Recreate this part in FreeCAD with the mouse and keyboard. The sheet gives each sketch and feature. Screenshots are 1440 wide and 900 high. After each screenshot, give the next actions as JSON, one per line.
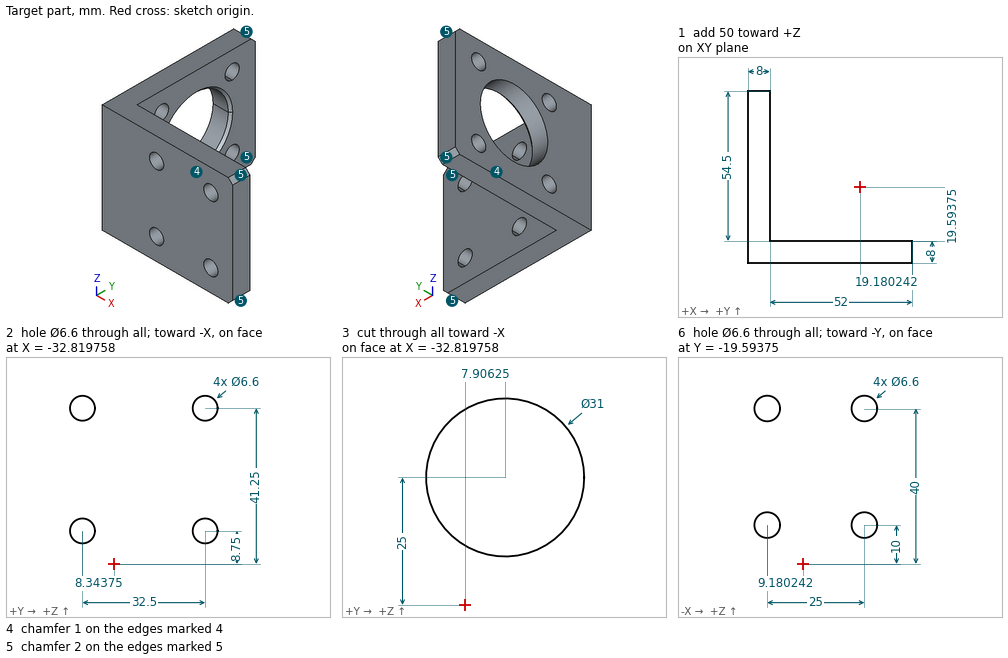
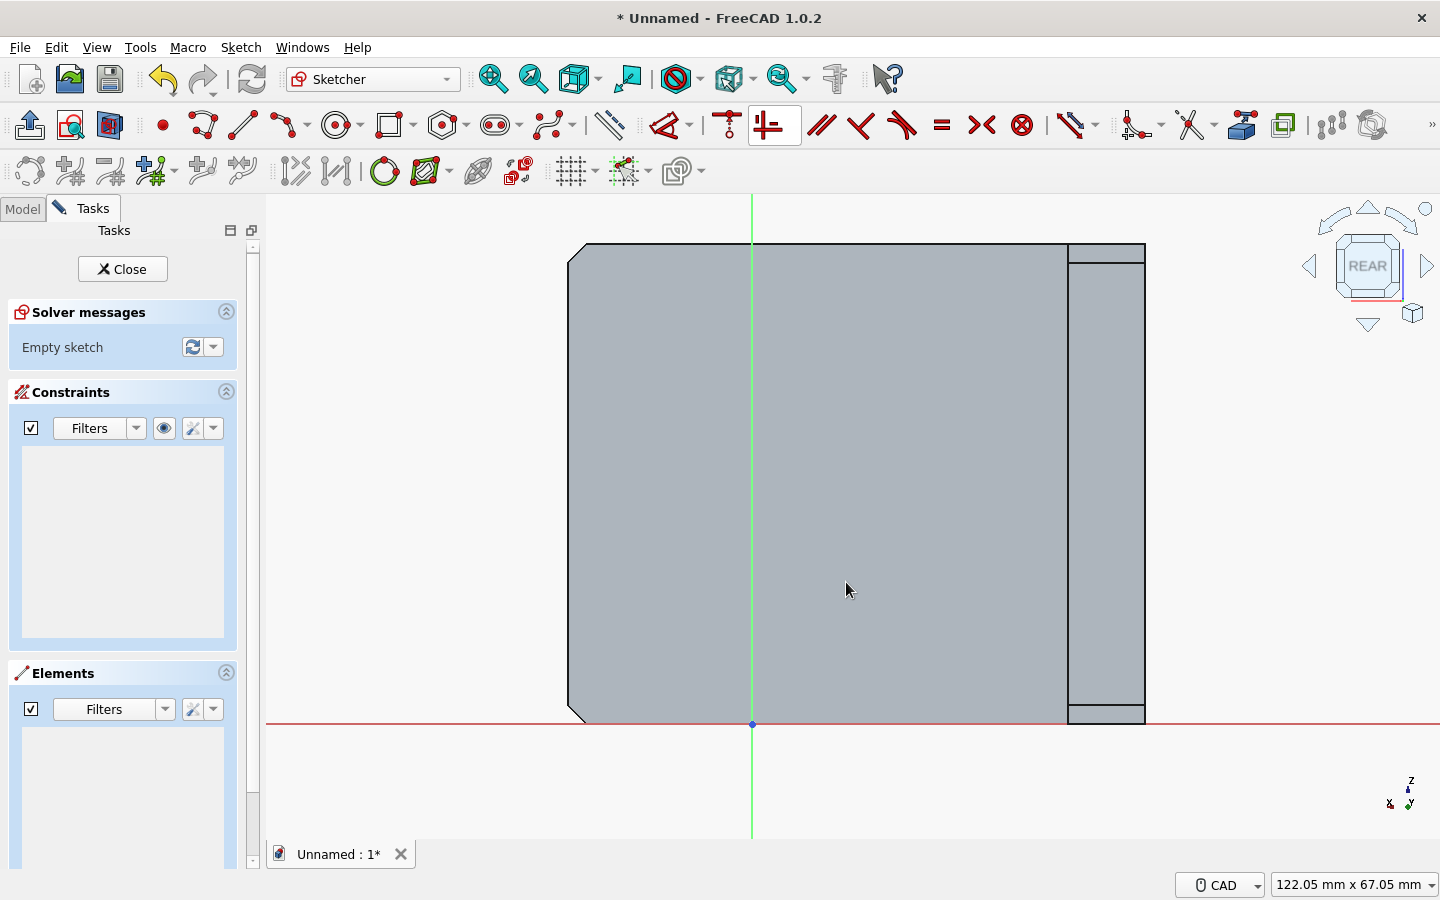
{"action": "left_click", "coordinate": [336, 126]}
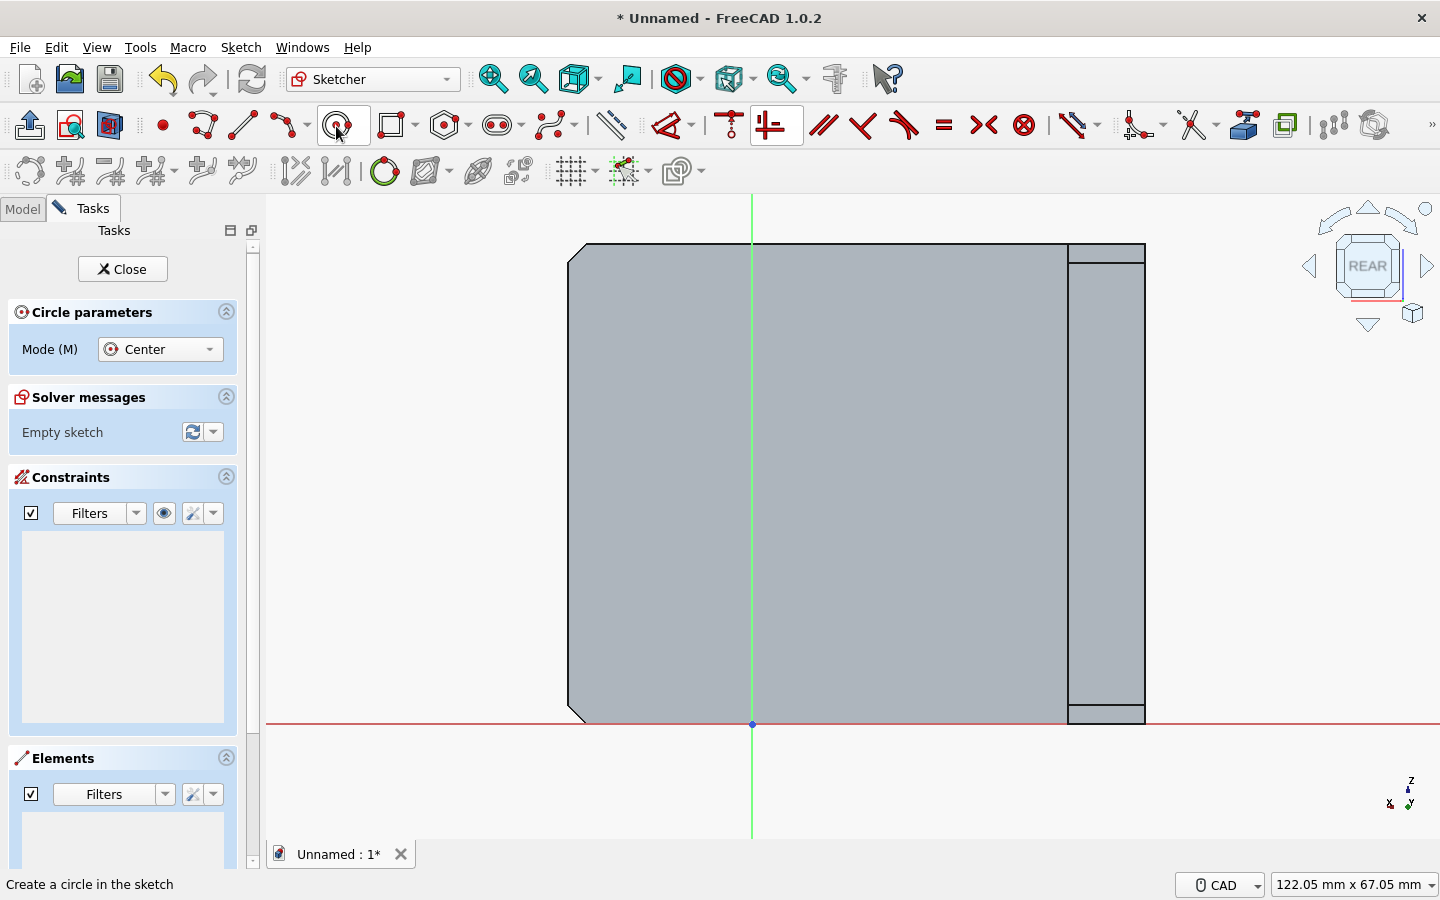
{"action": "left_click", "coordinate": [904, 340]}
{"action": "mouse_move", "coordinate": [927, 317]}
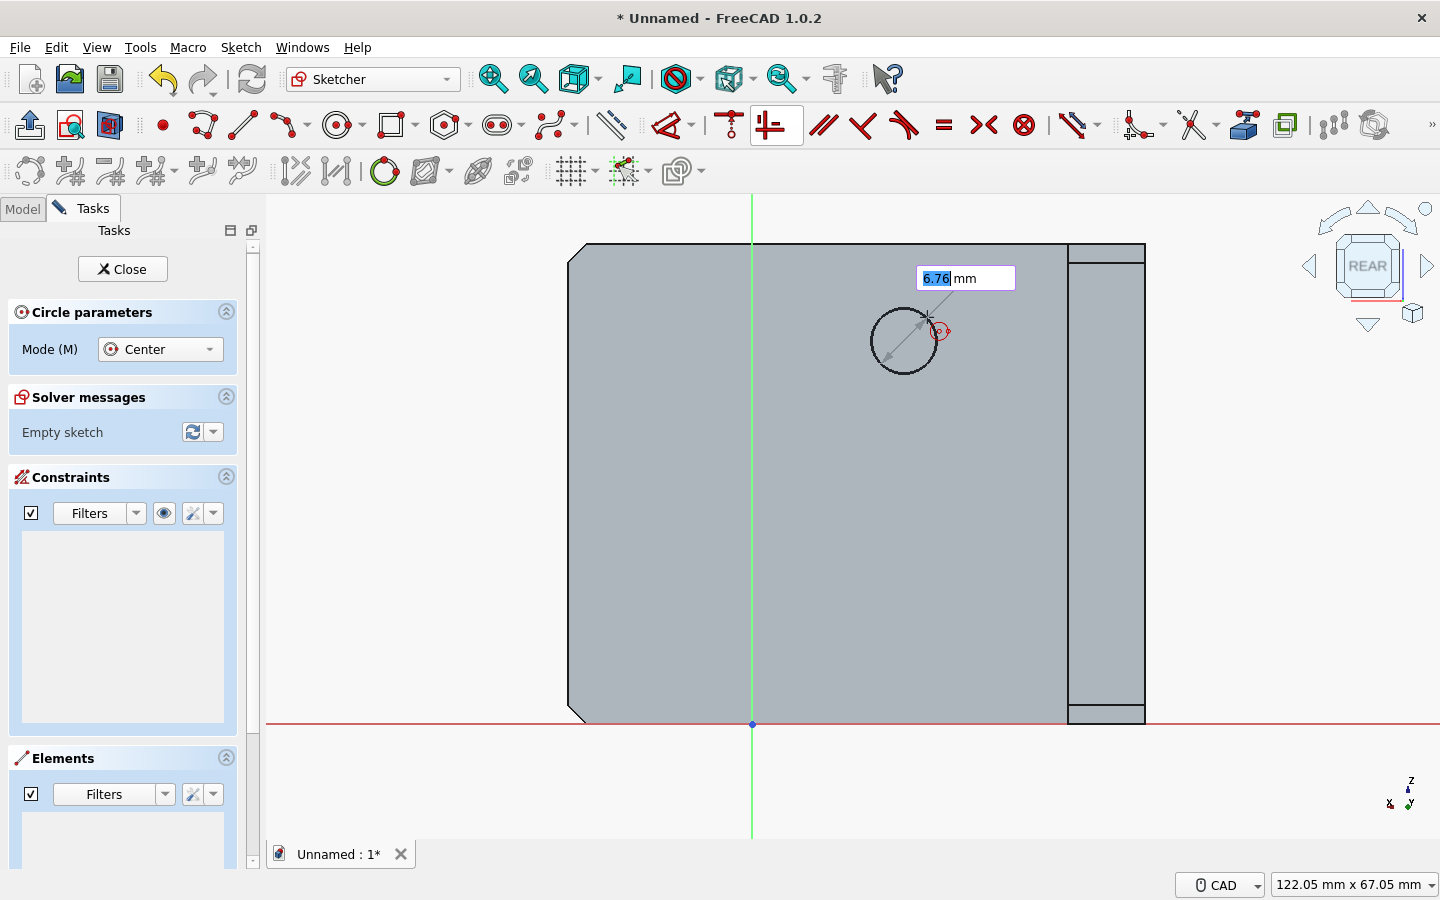
{"action": "type", "text": "6.6"}
{"action": "key", "text": "Return"}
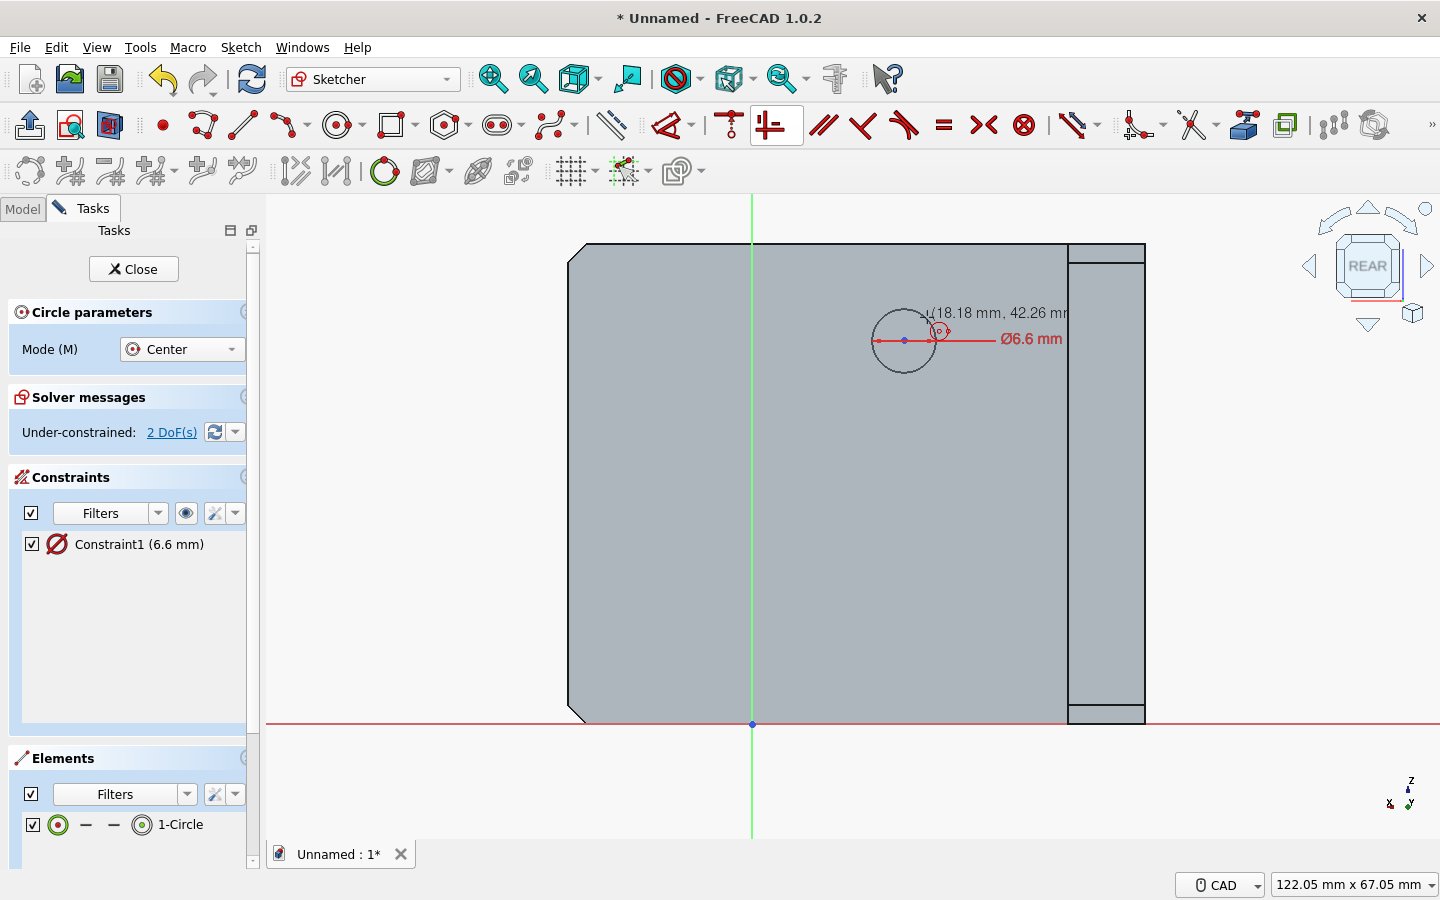
{"action": "left_click", "coordinate": [904, 628]}
{"action": "mouse_move", "coordinate": [927, 606]}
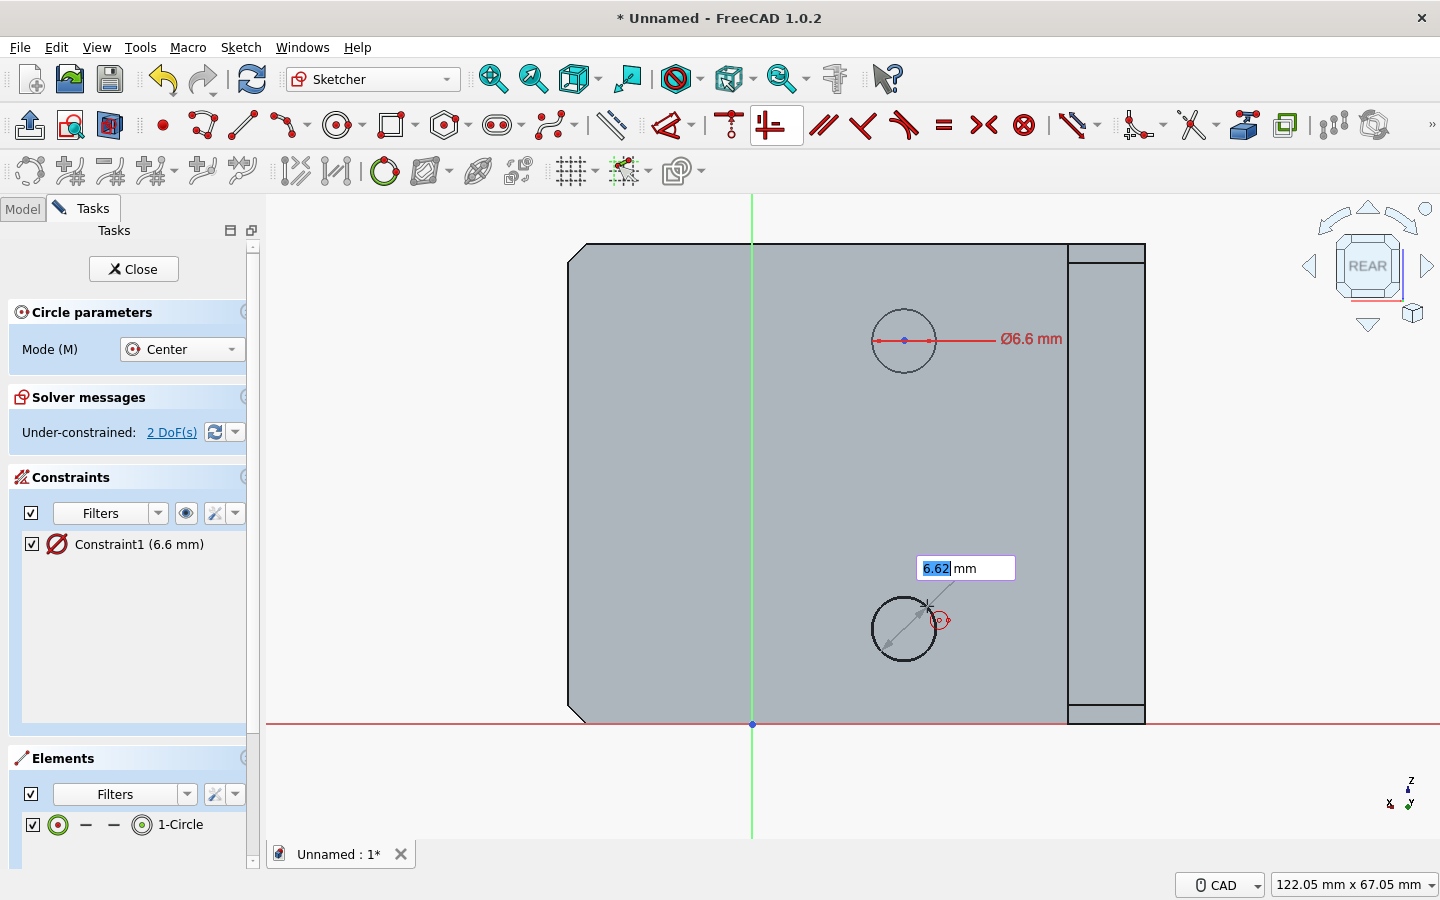
{"action": "type", "text": "6.6"}
{"action": "key", "text": "Return"}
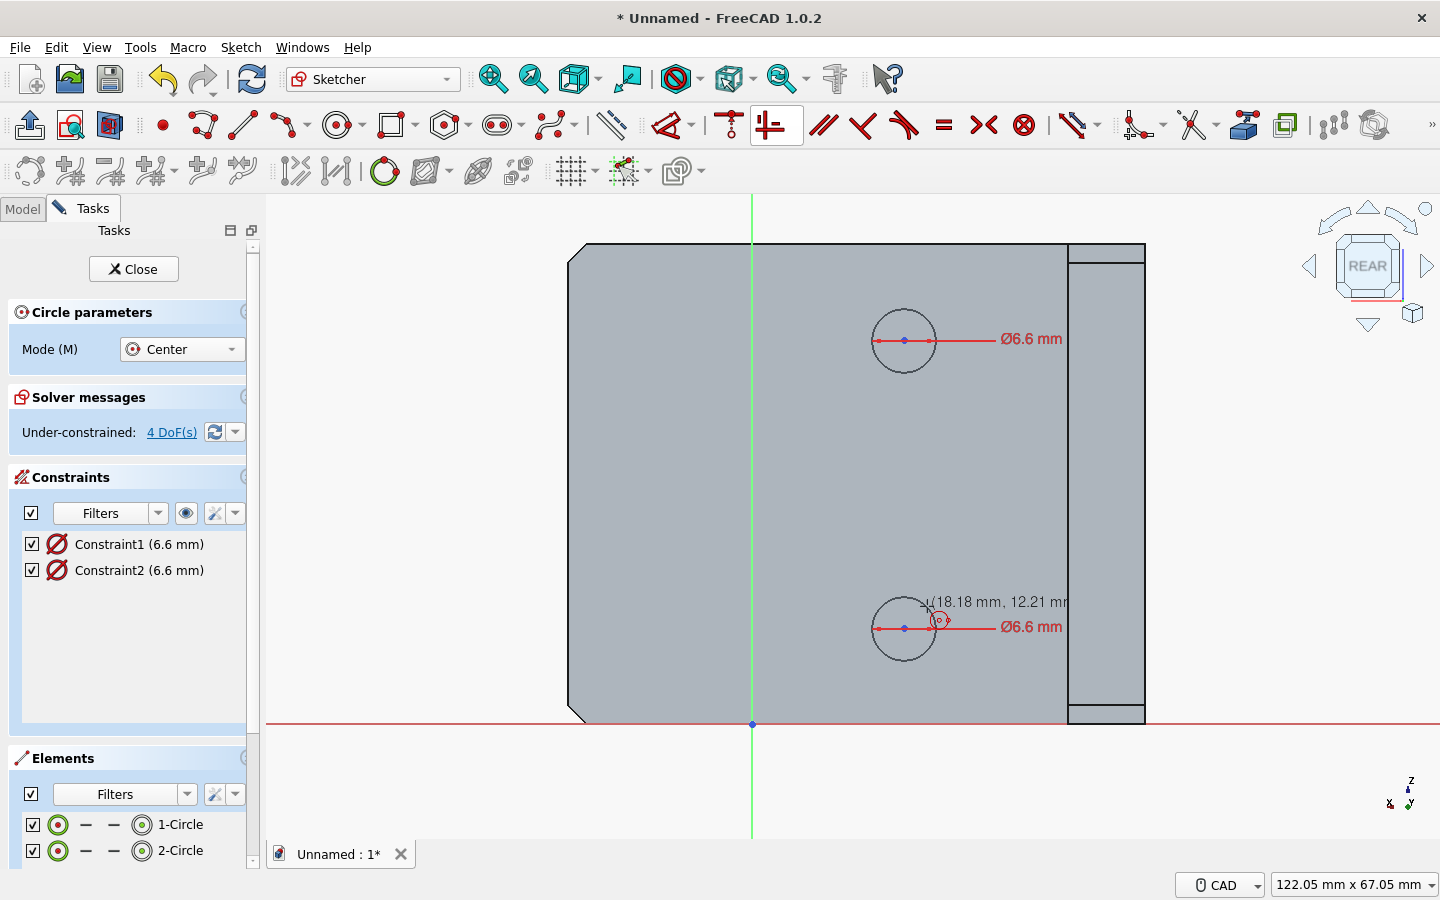
{"action": "left_click", "coordinate": [664, 628]}
{"action": "mouse_move", "coordinate": [686, 606]}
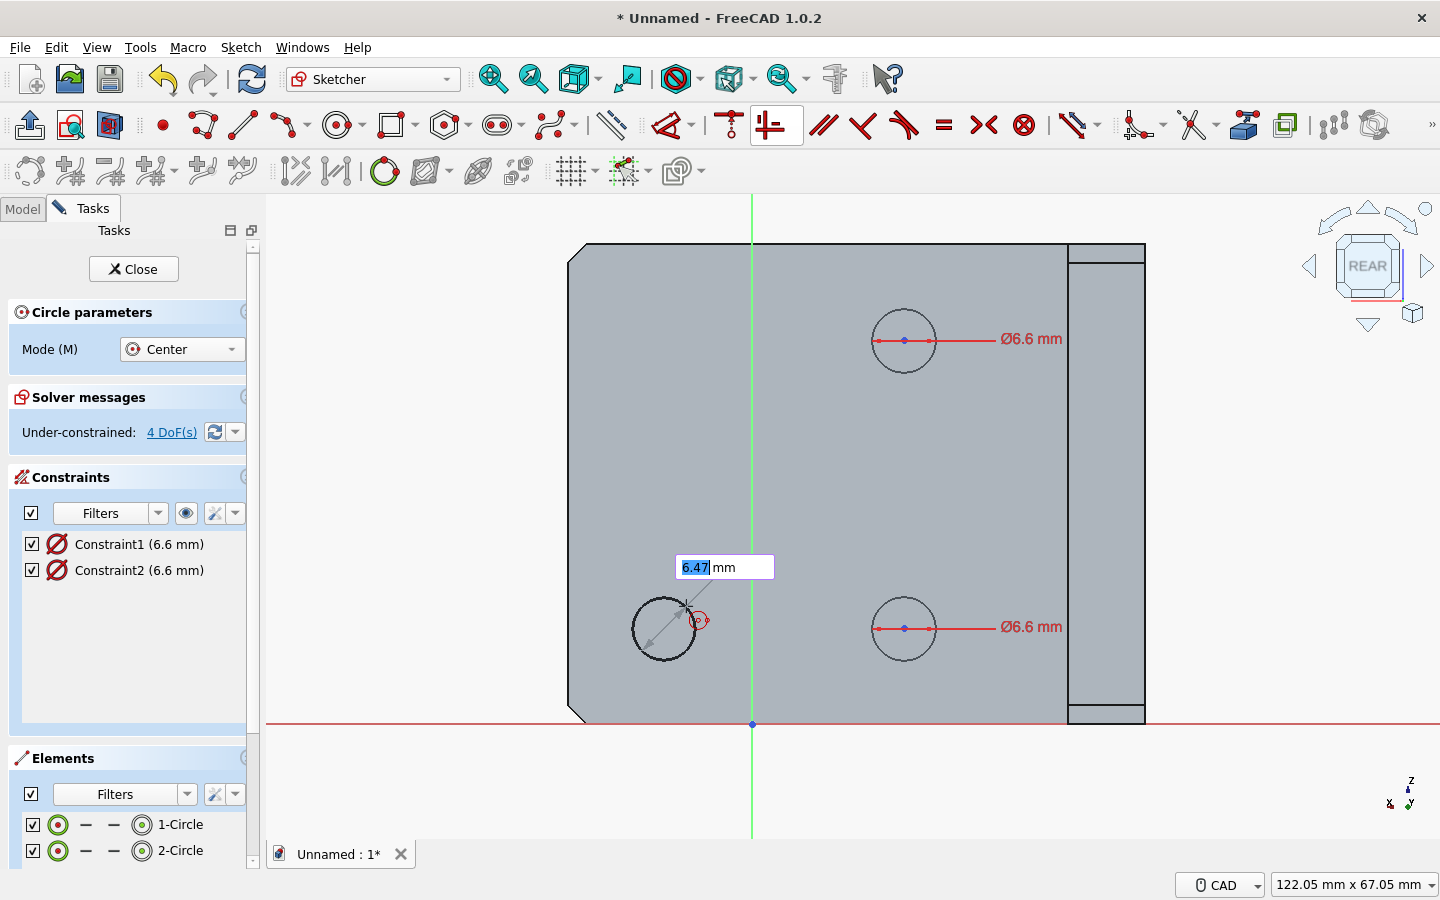
{"action": "type", "text": "6.6"}
{"action": "key", "text": "Return"}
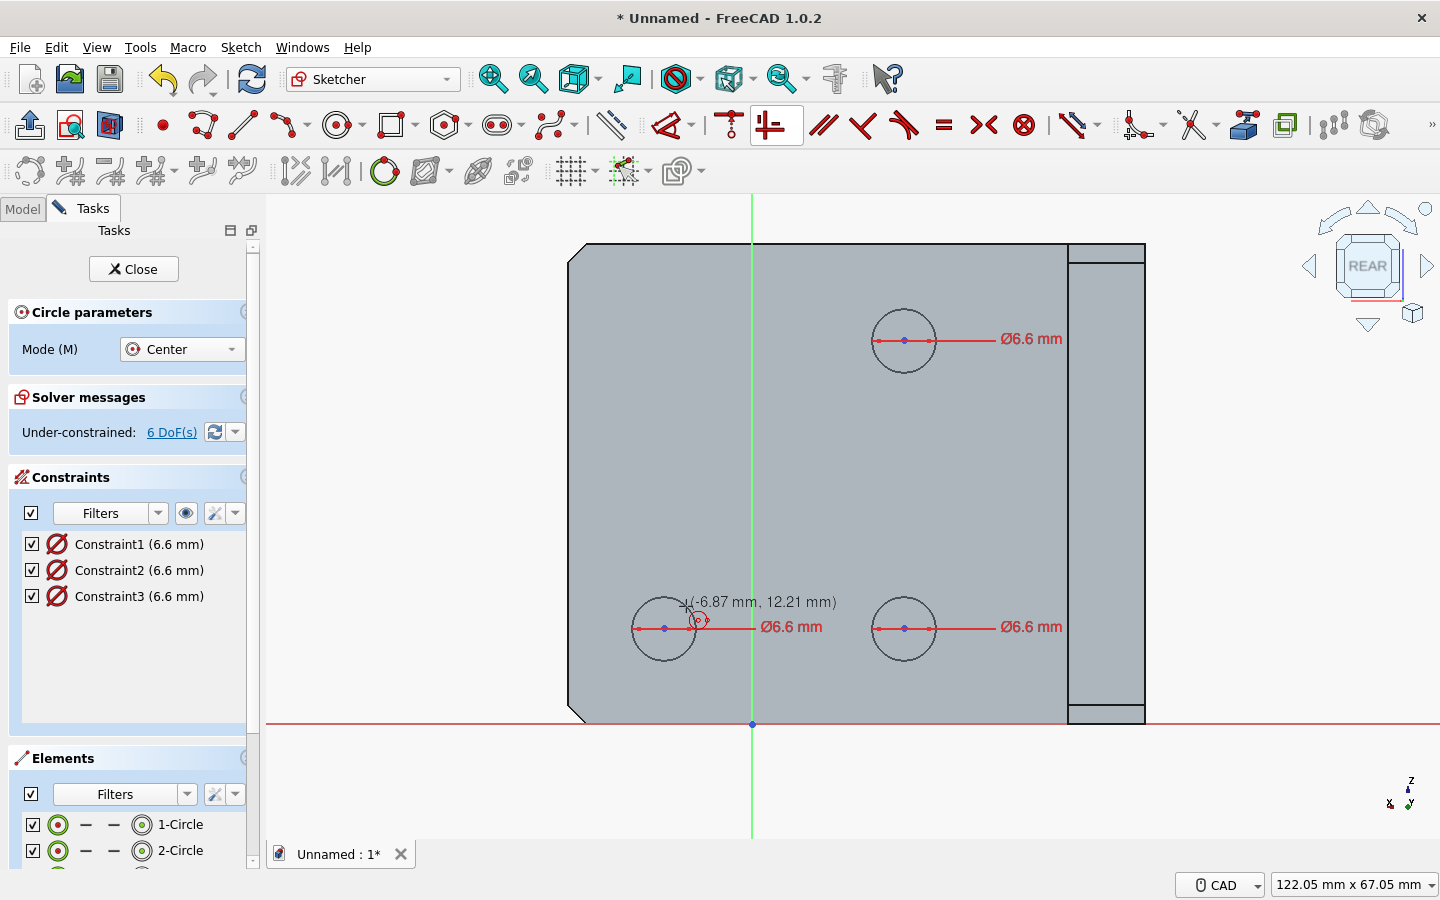
{"action": "left_click", "coordinate": [664, 340]}
{"action": "mouse_move", "coordinate": [686, 317]}